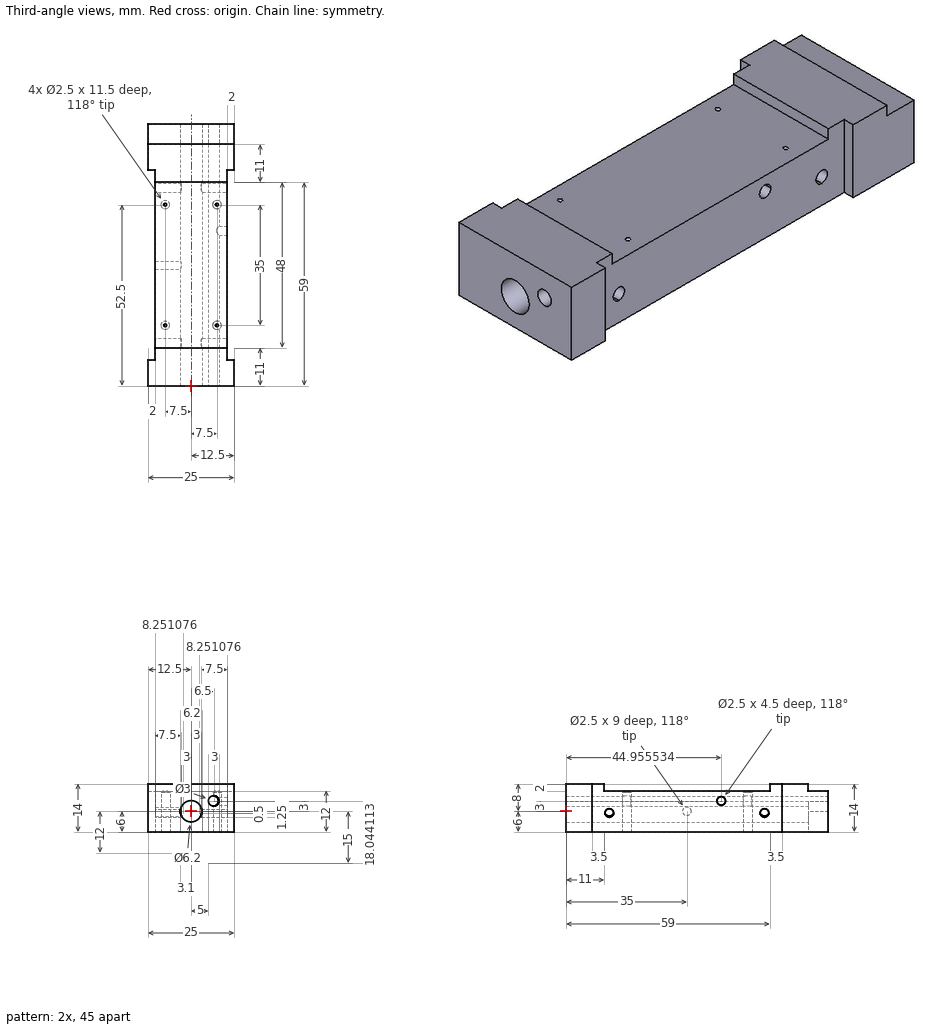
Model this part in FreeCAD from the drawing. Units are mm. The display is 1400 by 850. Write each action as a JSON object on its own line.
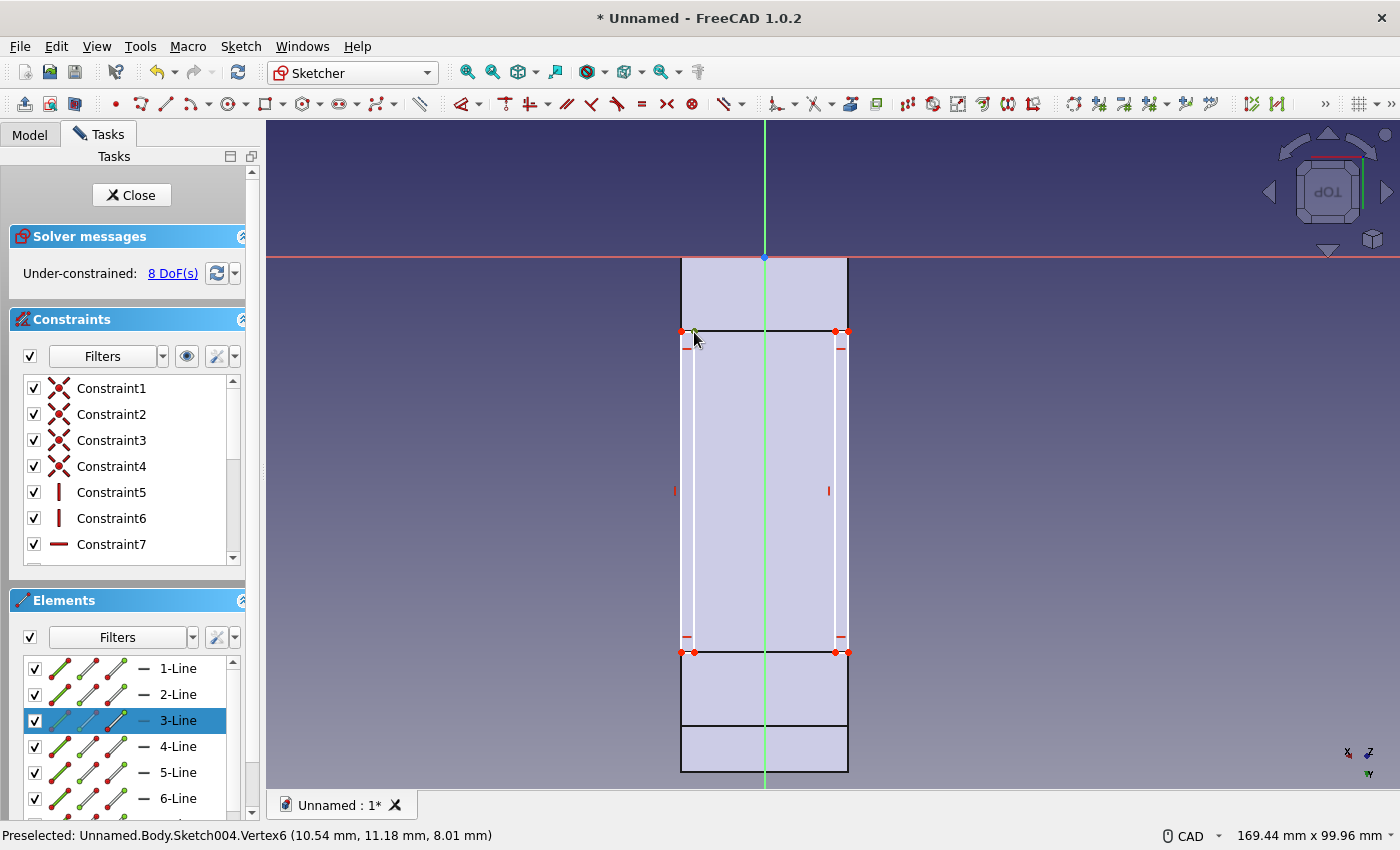
{"action": "left_click", "coordinate": [835, 332]}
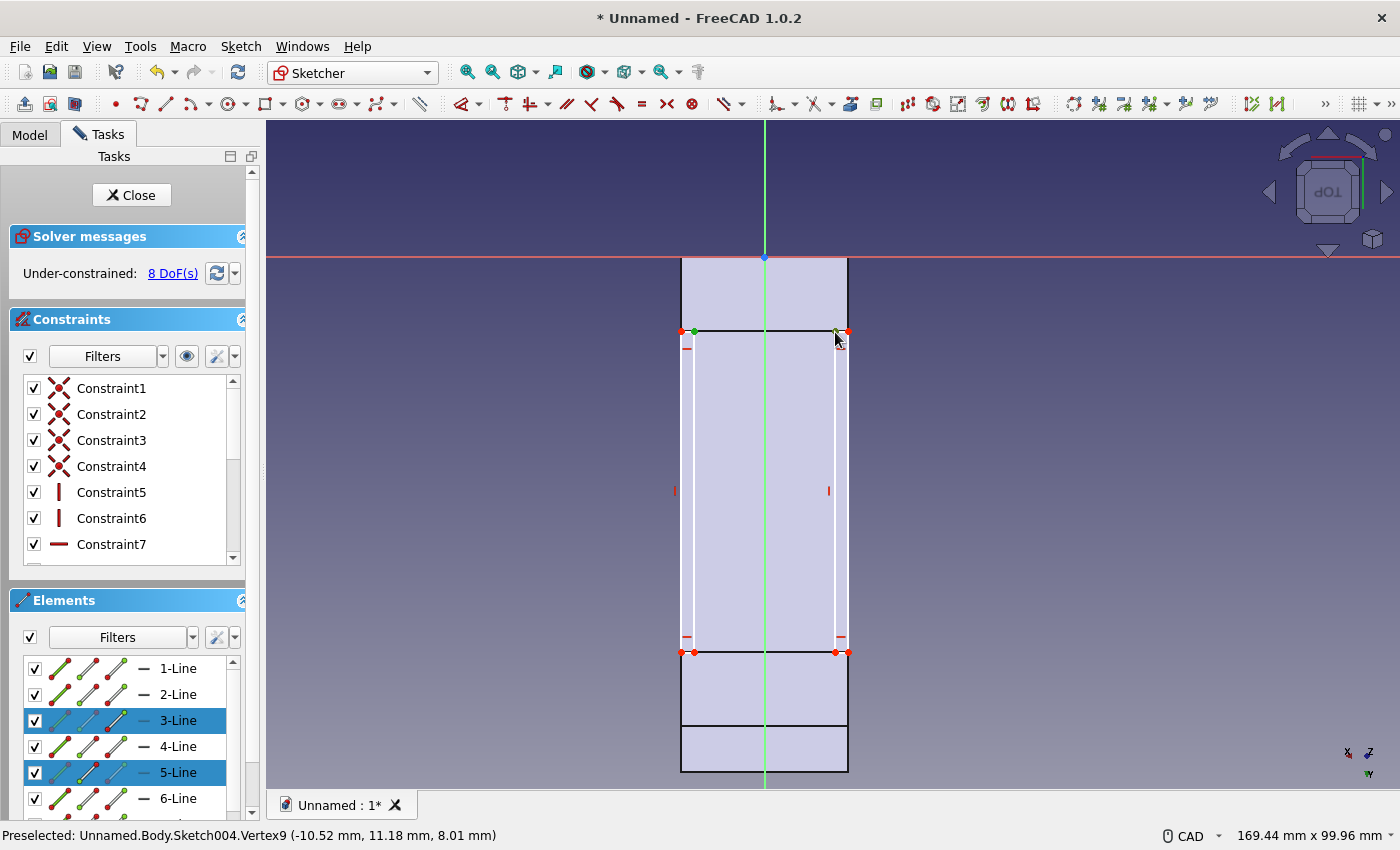
{"action": "left_click", "coordinate": [765, 717]}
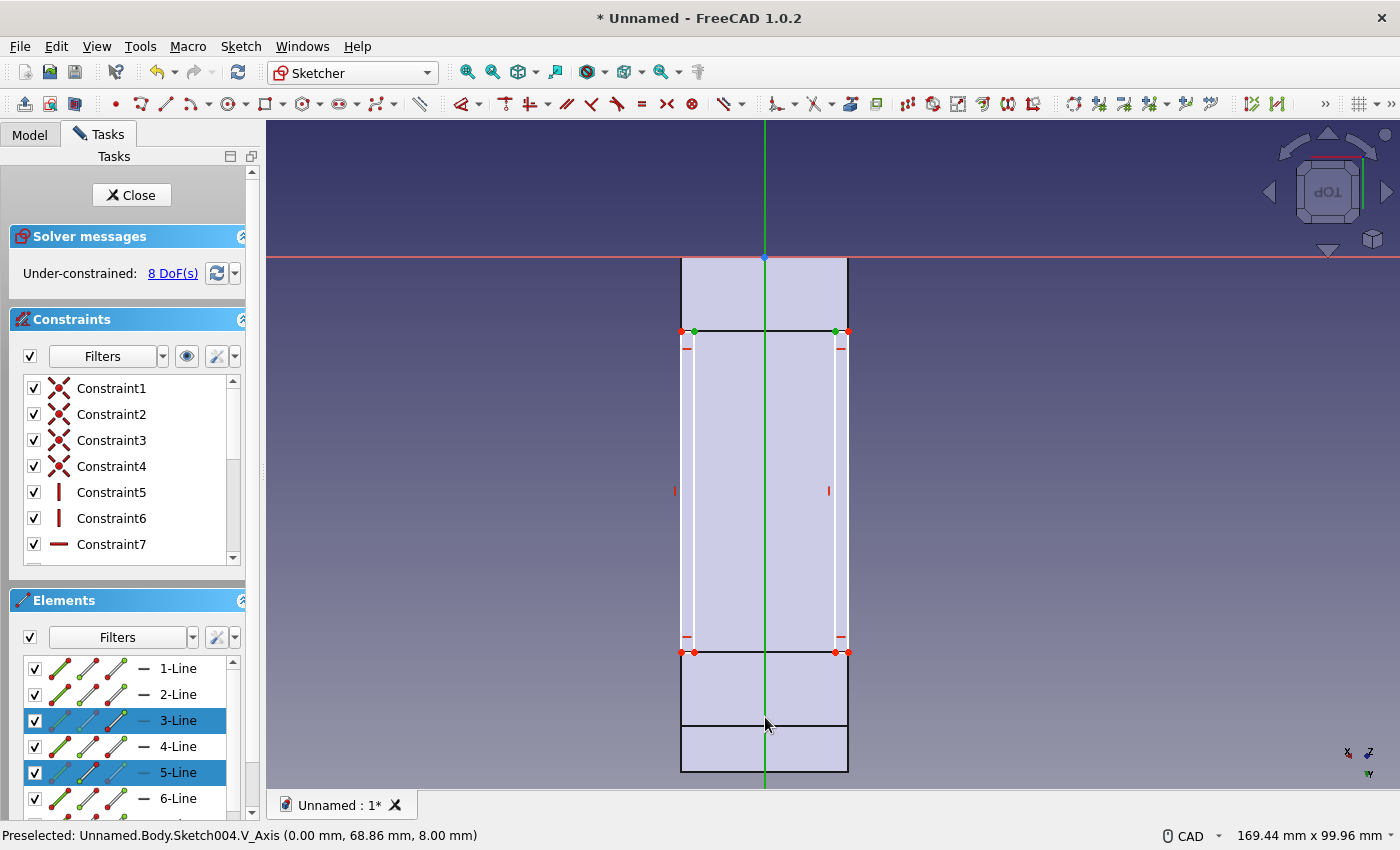
{"action": "left_click", "coordinate": [667, 104]}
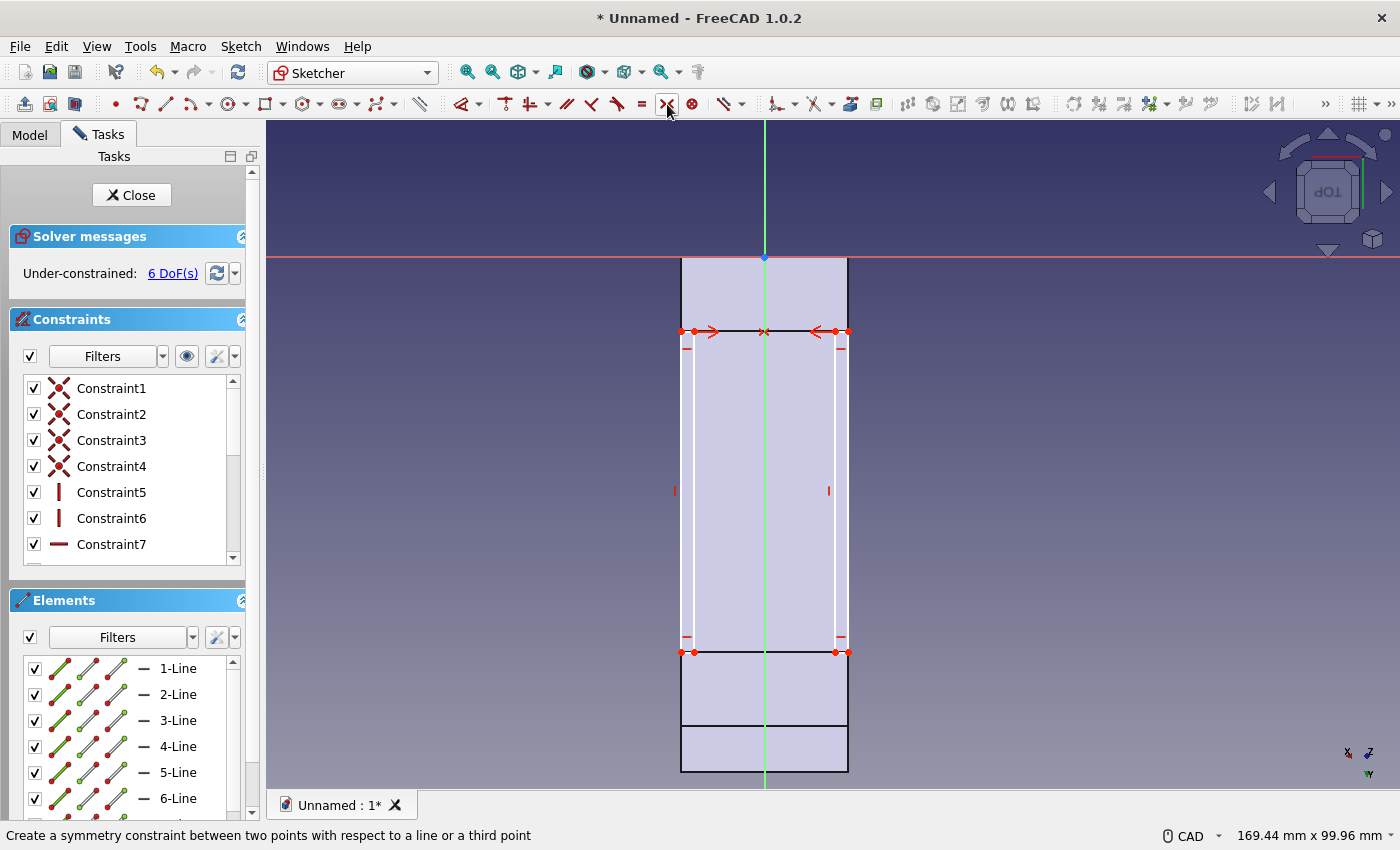
{"action": "left_click", "coordinate": [681, 653]}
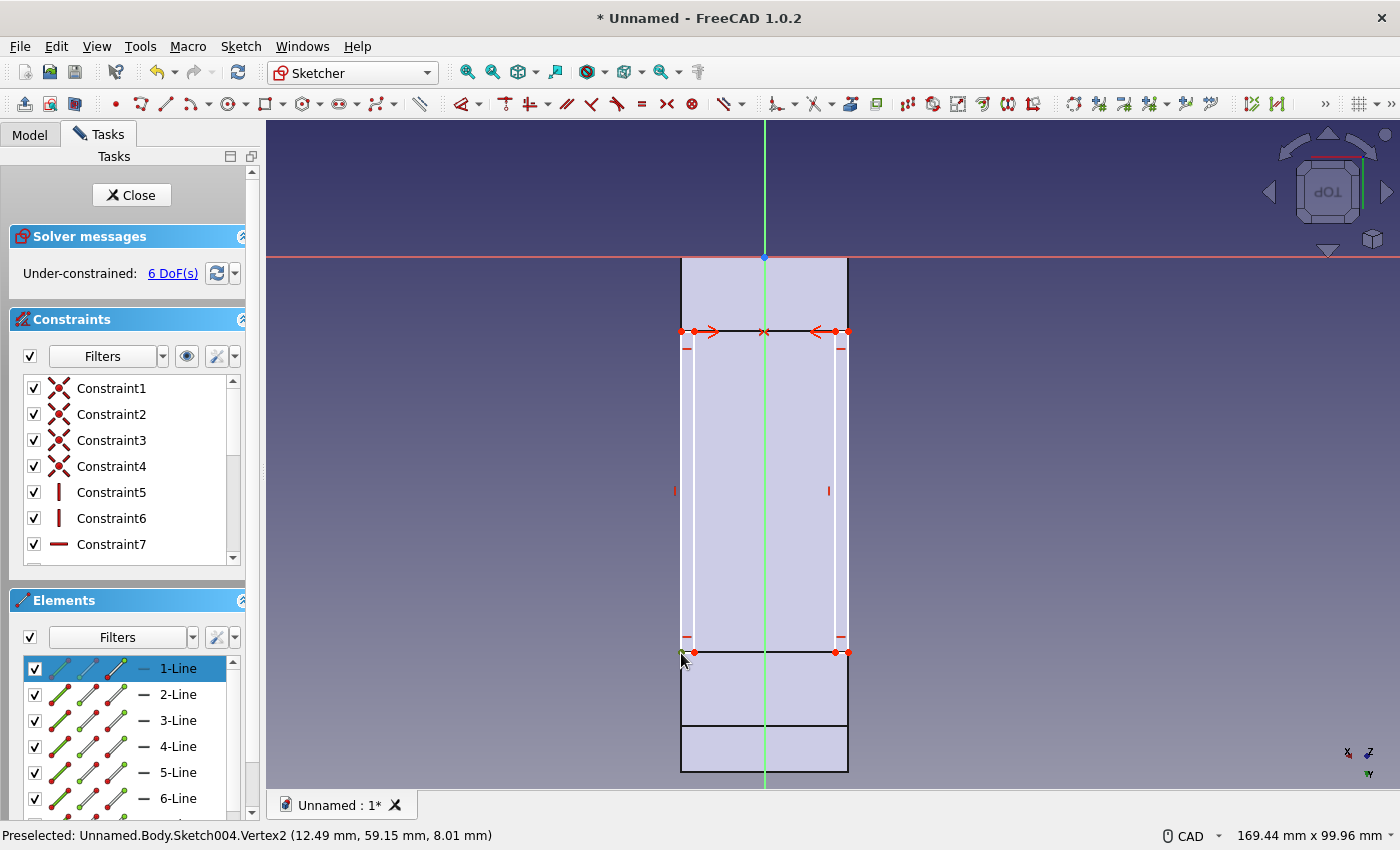
{"action": "left_click", "coordinate": [848, 653]}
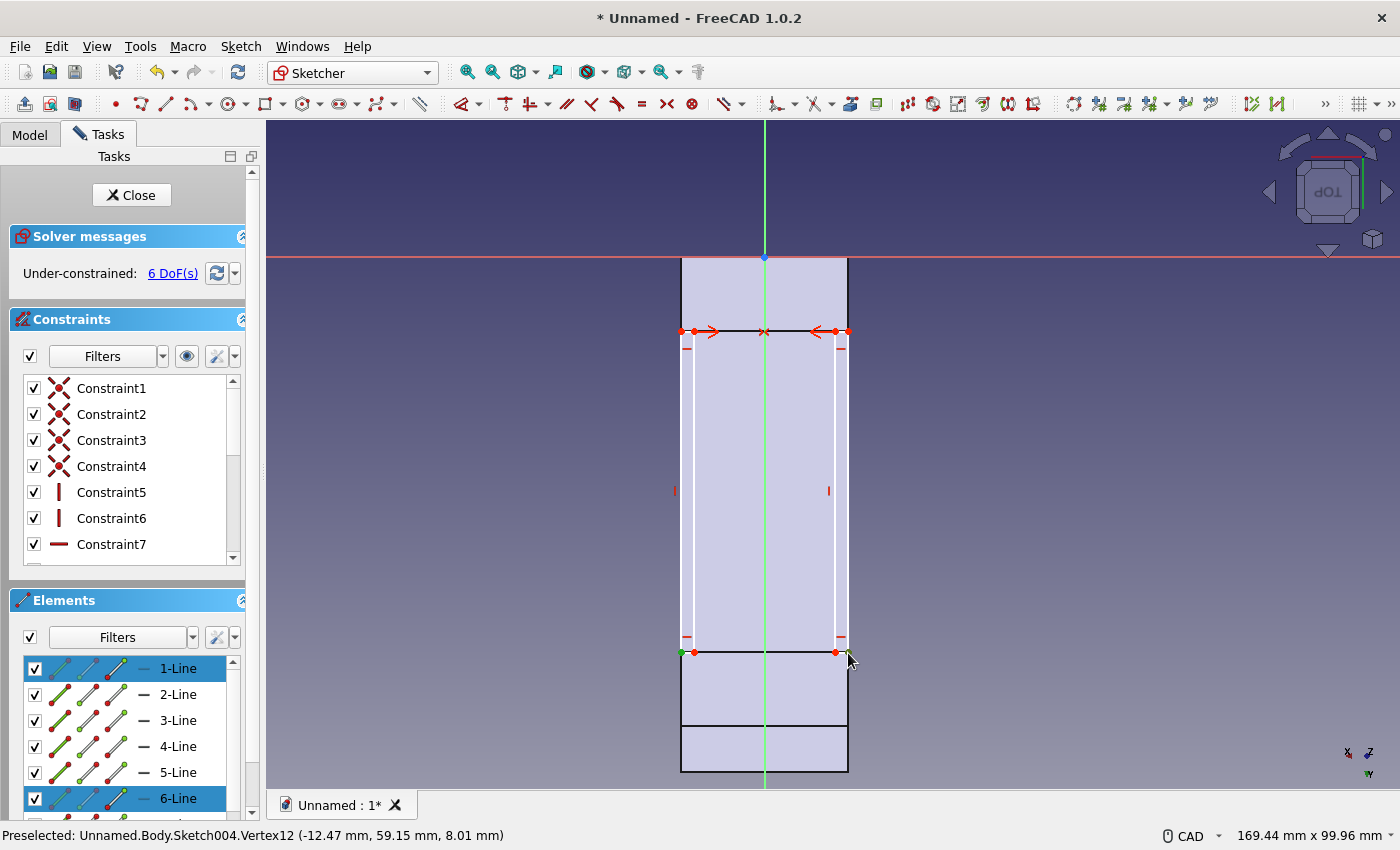
{"action": "left_click", "coordinate": [765, 717]}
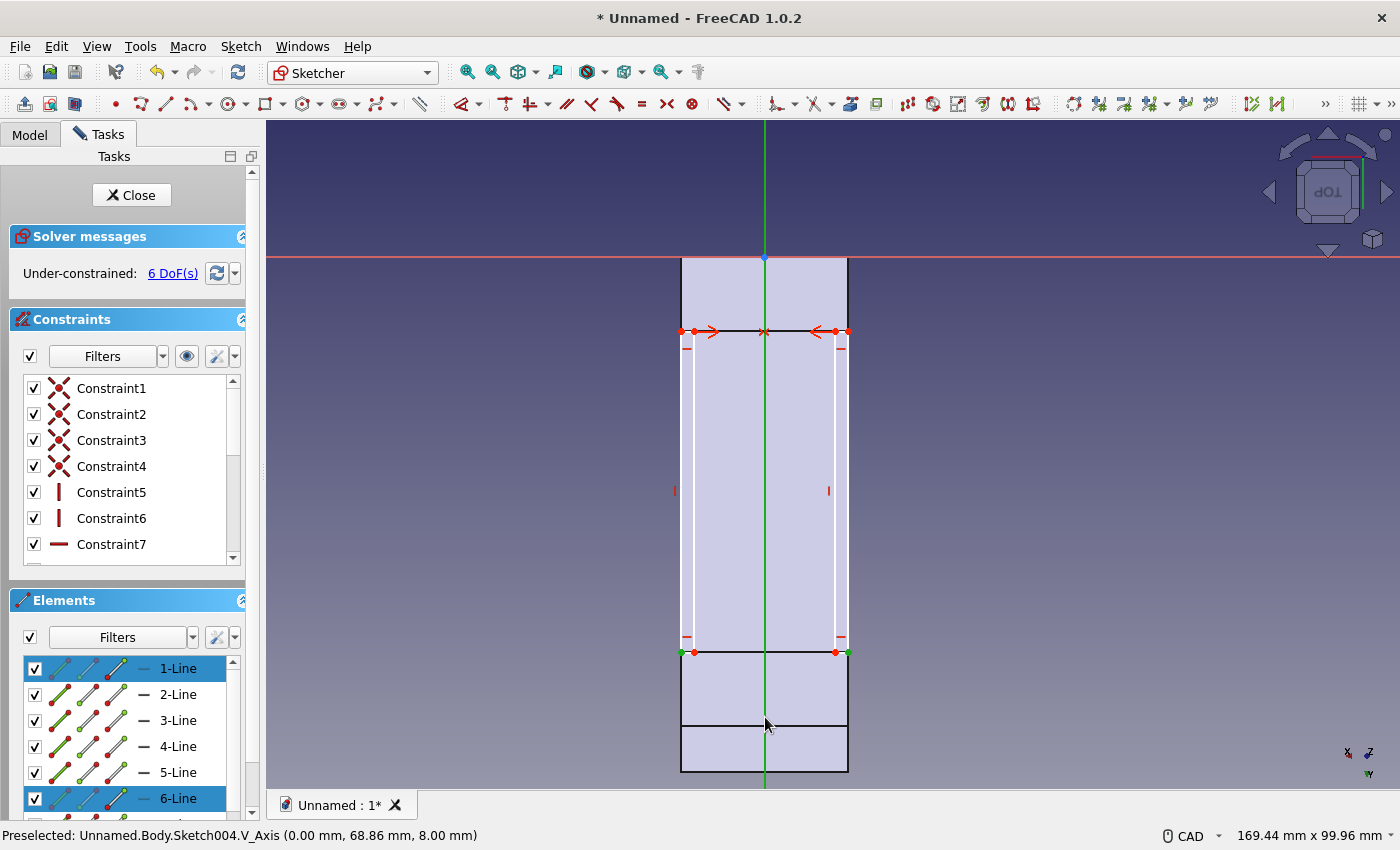
{"action": "left_click", "coordinate": [667, 104]}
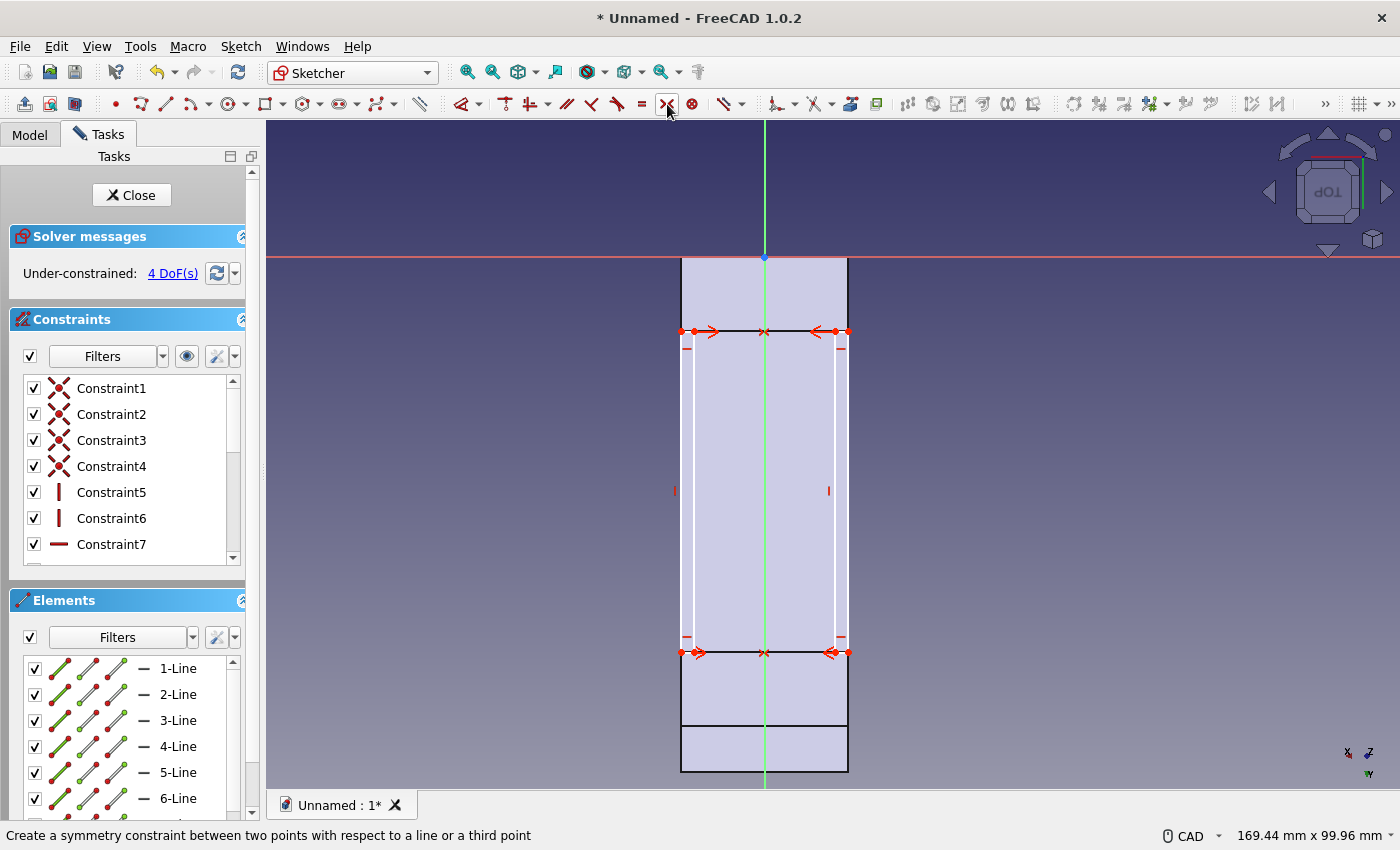
{"action": "left_click", "coordinate": [460, 104]}